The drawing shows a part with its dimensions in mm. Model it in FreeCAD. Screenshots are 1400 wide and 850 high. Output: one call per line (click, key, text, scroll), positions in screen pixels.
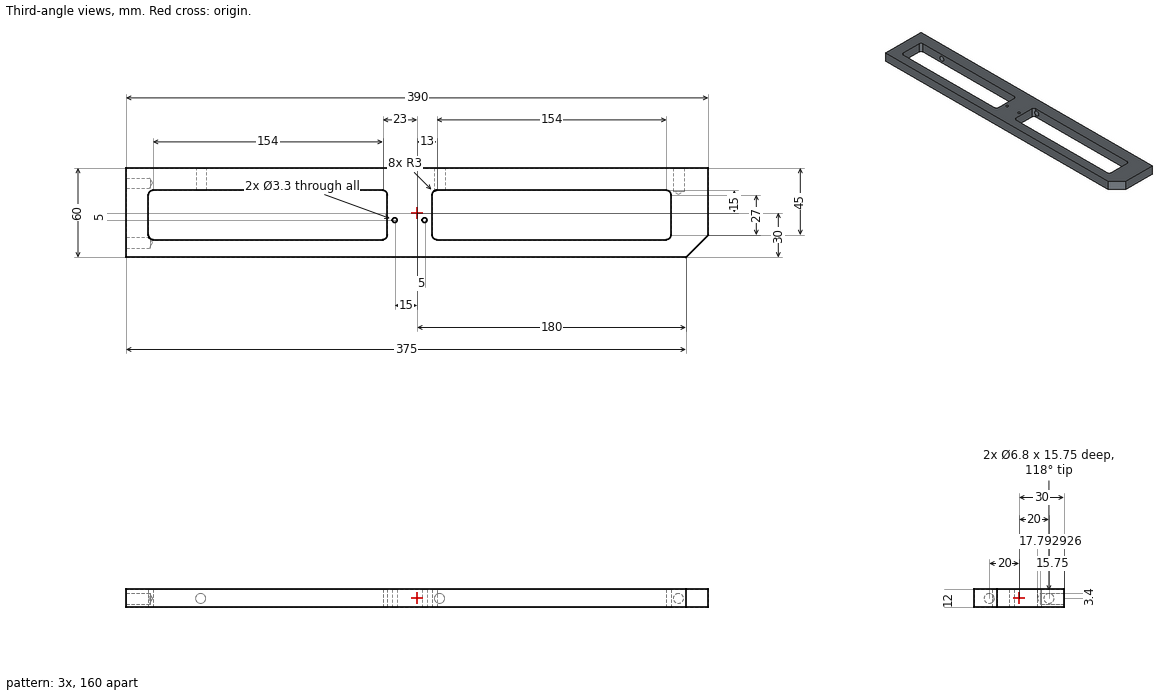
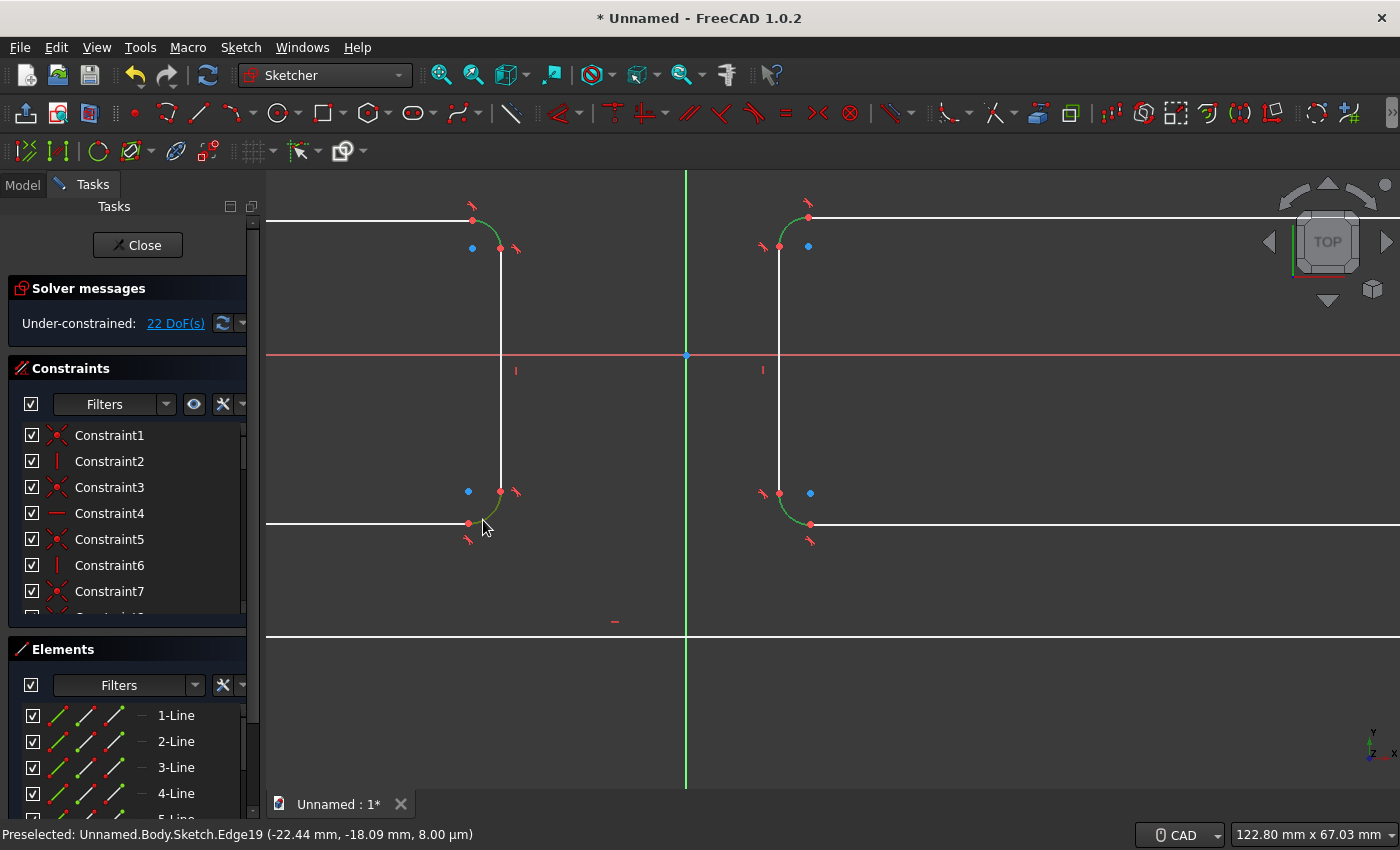
scroll(784, 511, down, 8)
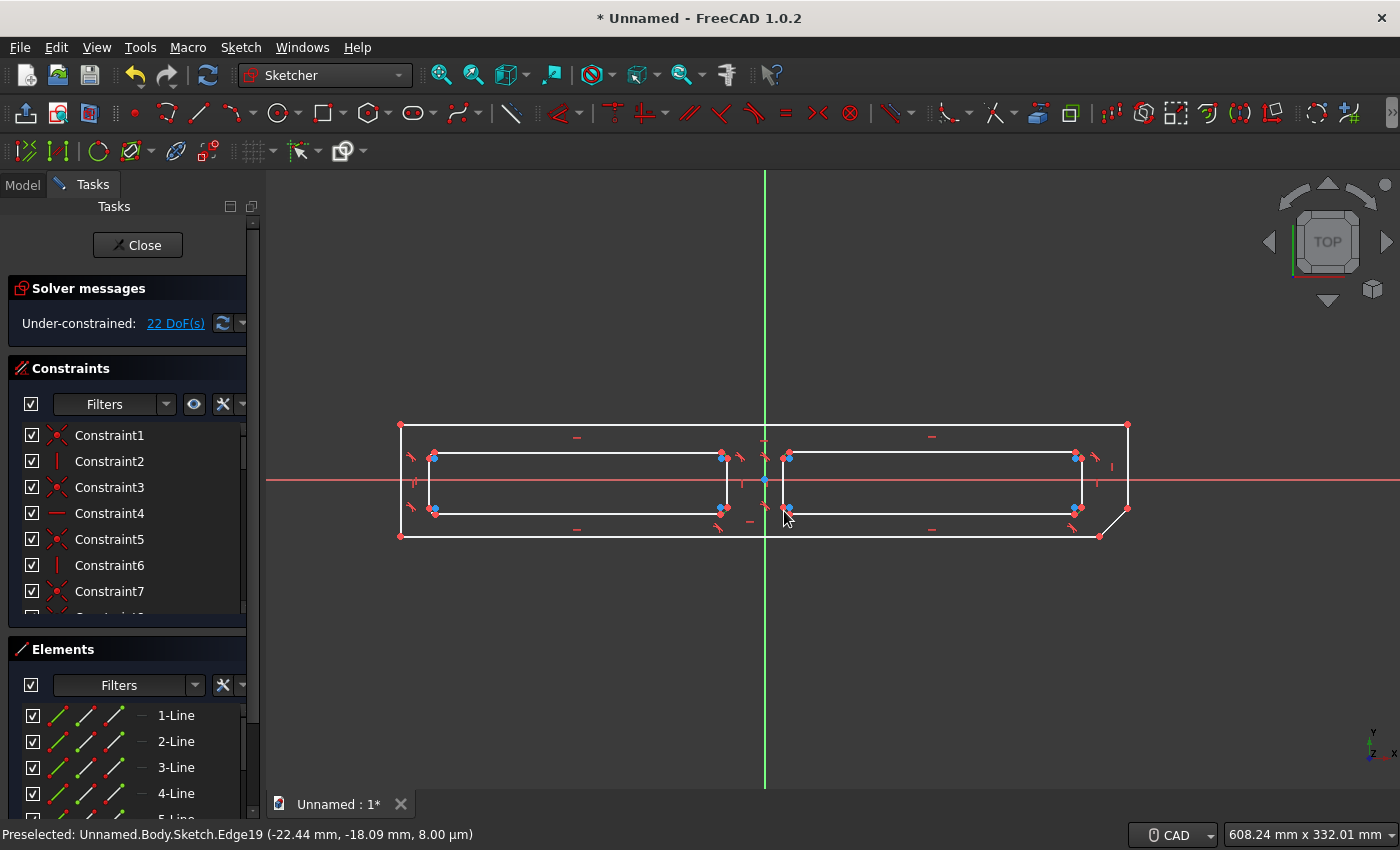
scroll(430, 511, up, 8)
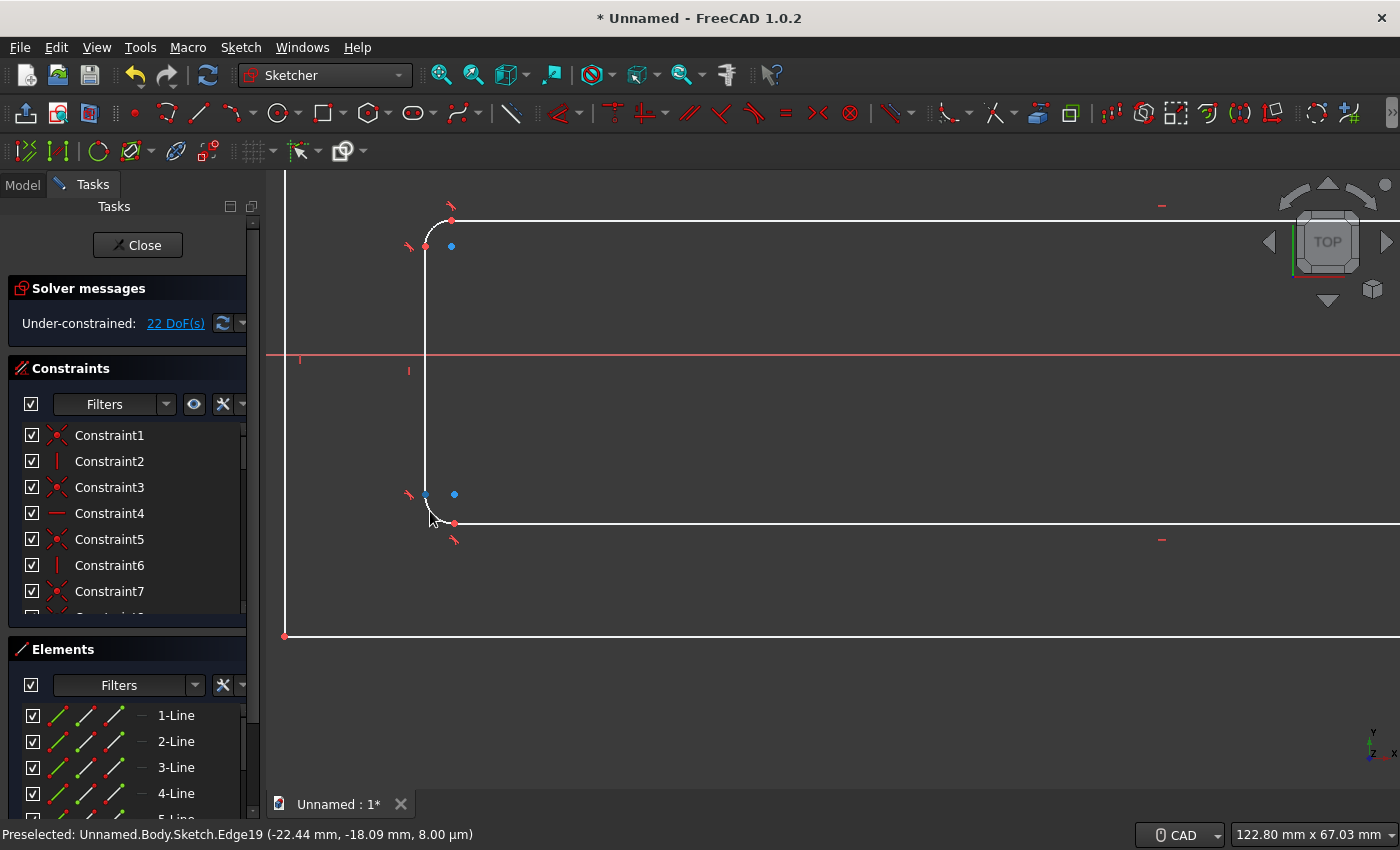
click(428, 508)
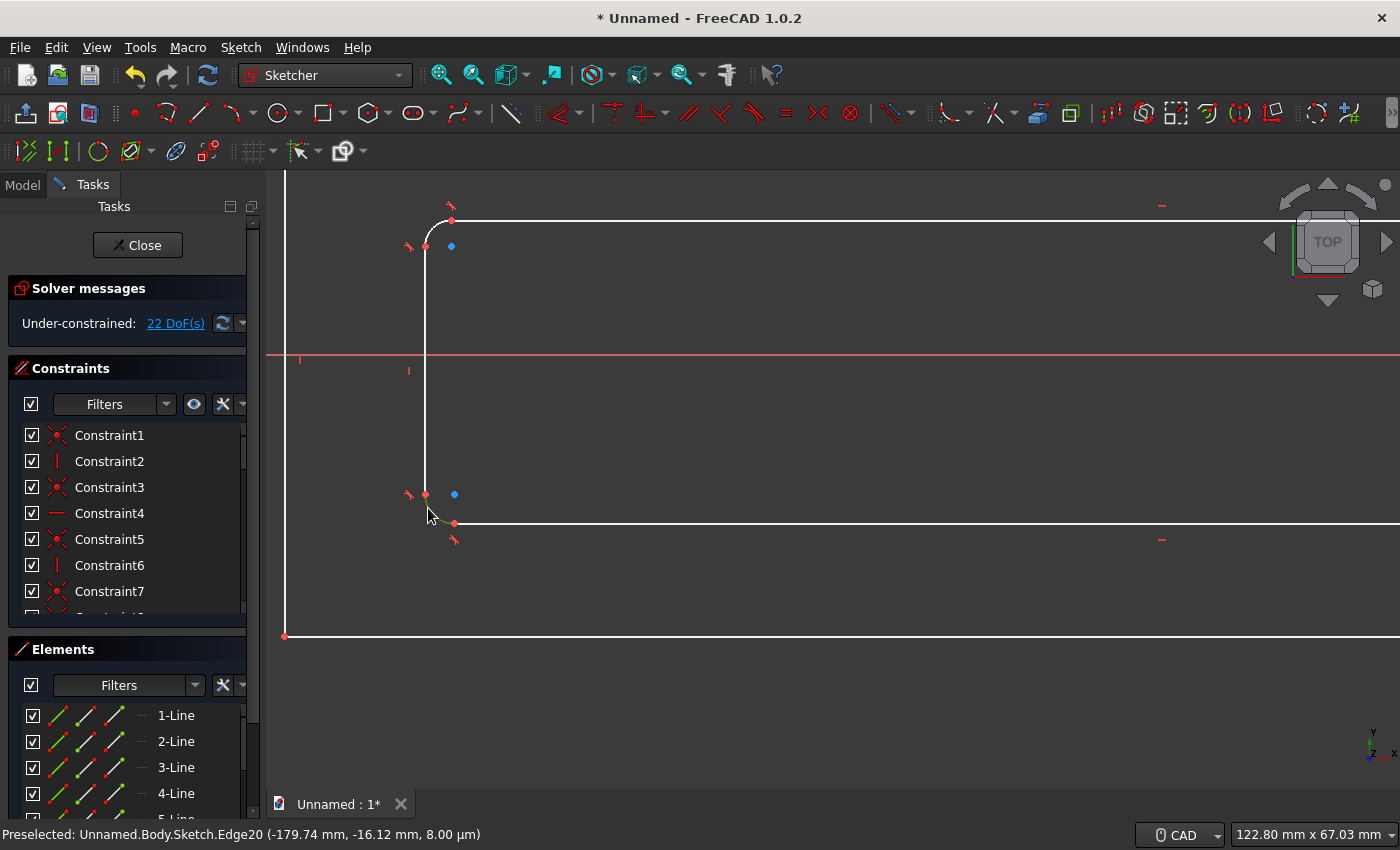
click(439, 223)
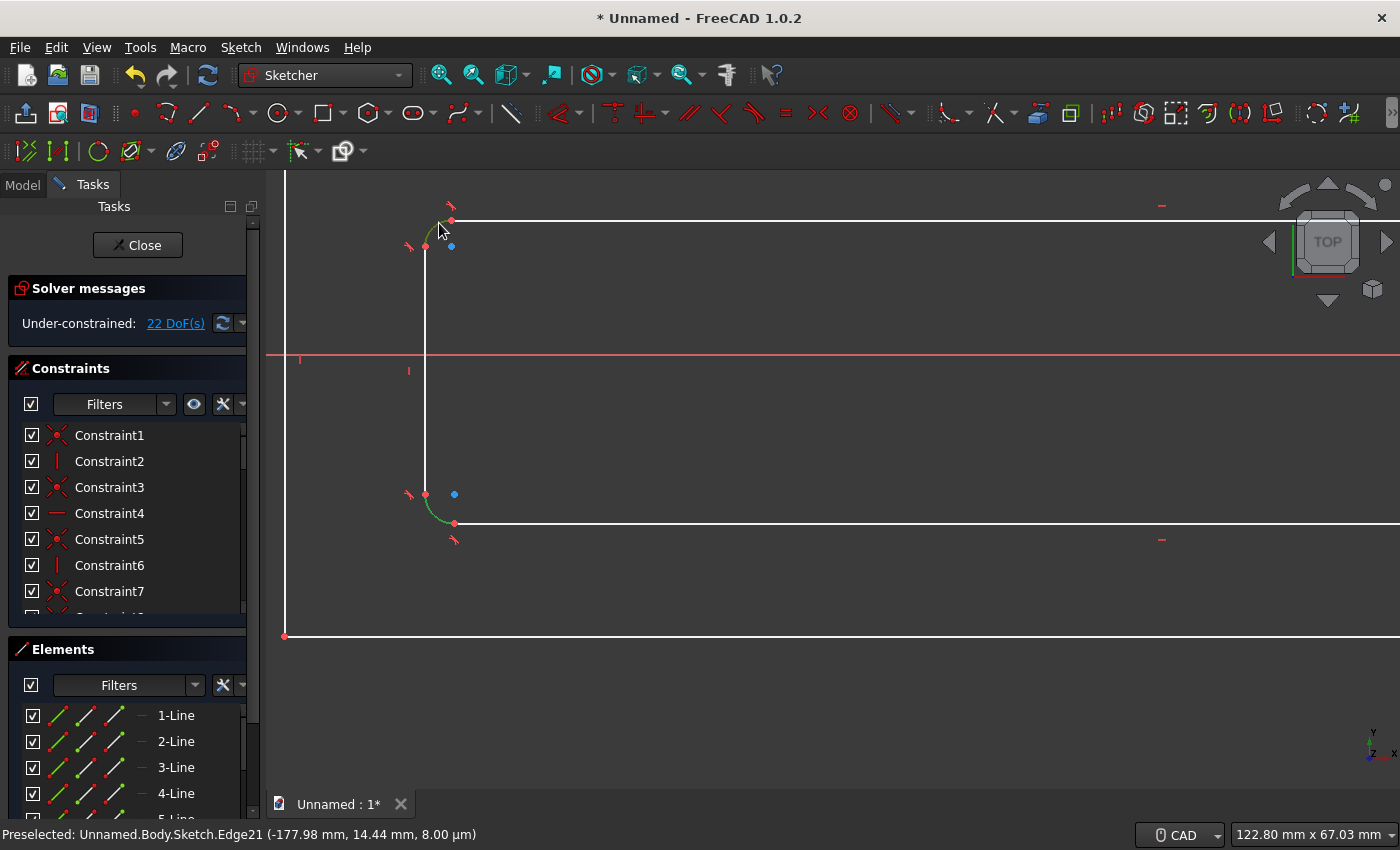
key(e)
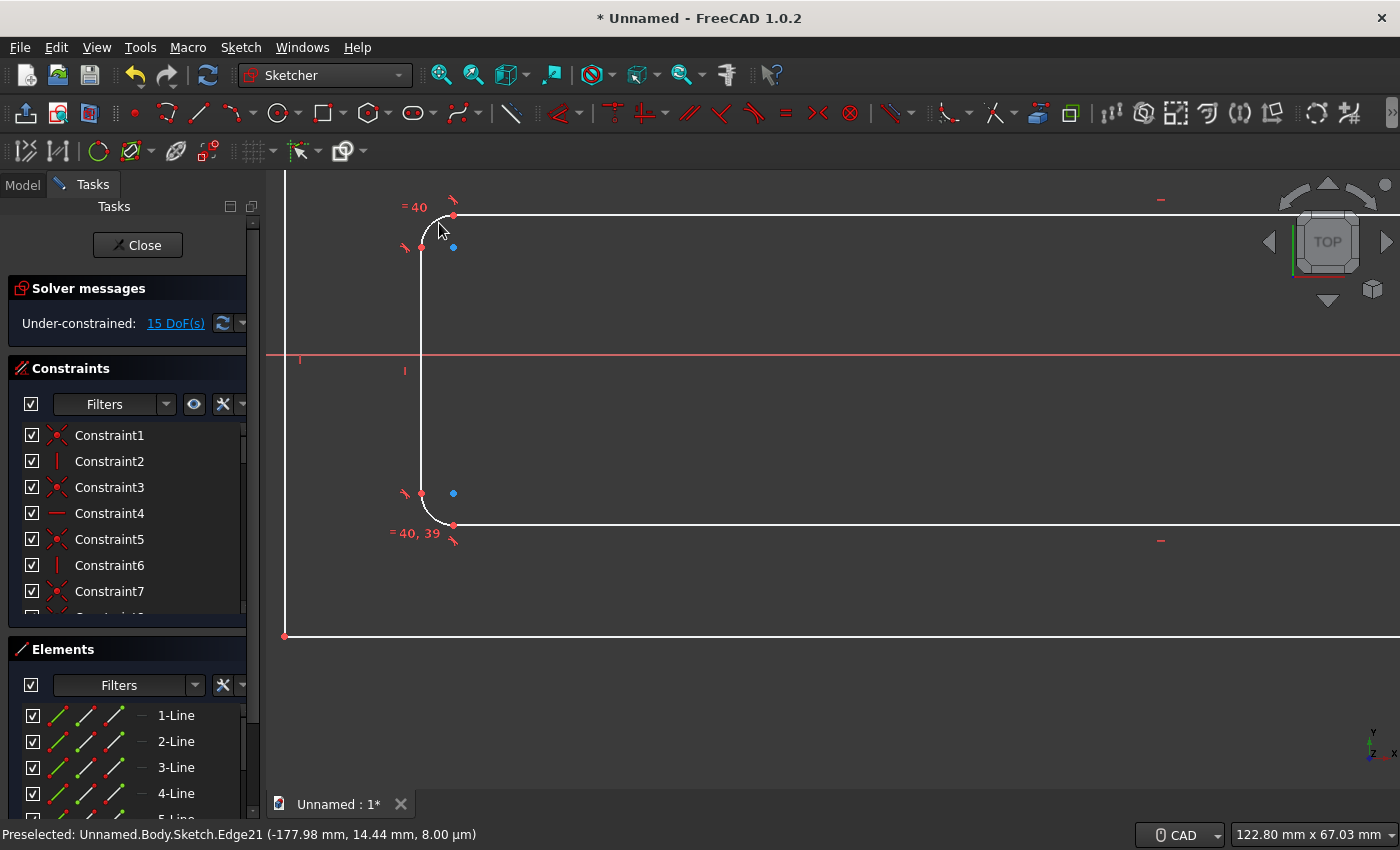
scroll(430, 511, down, 8)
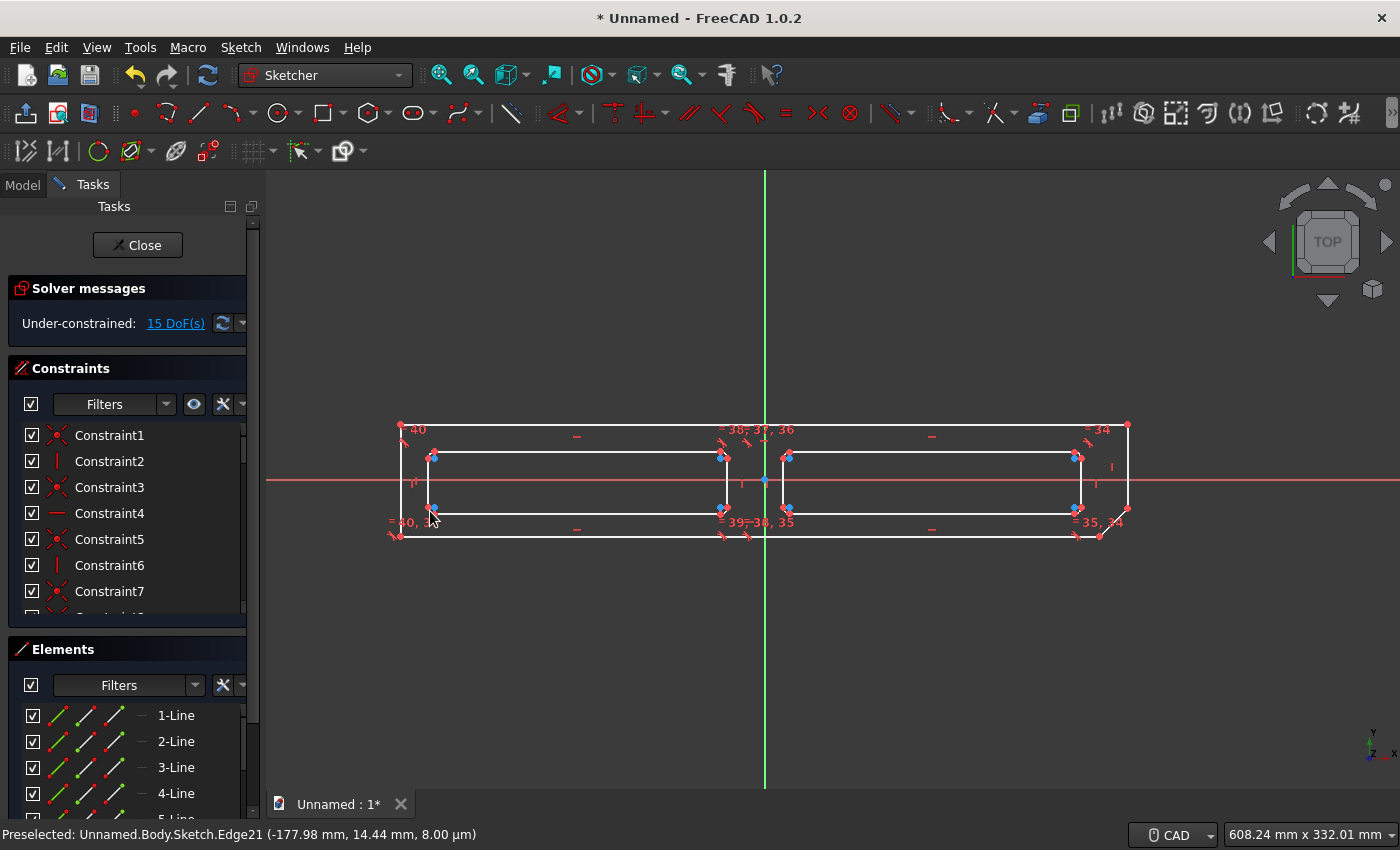
scroll(1081, 456, up, 10)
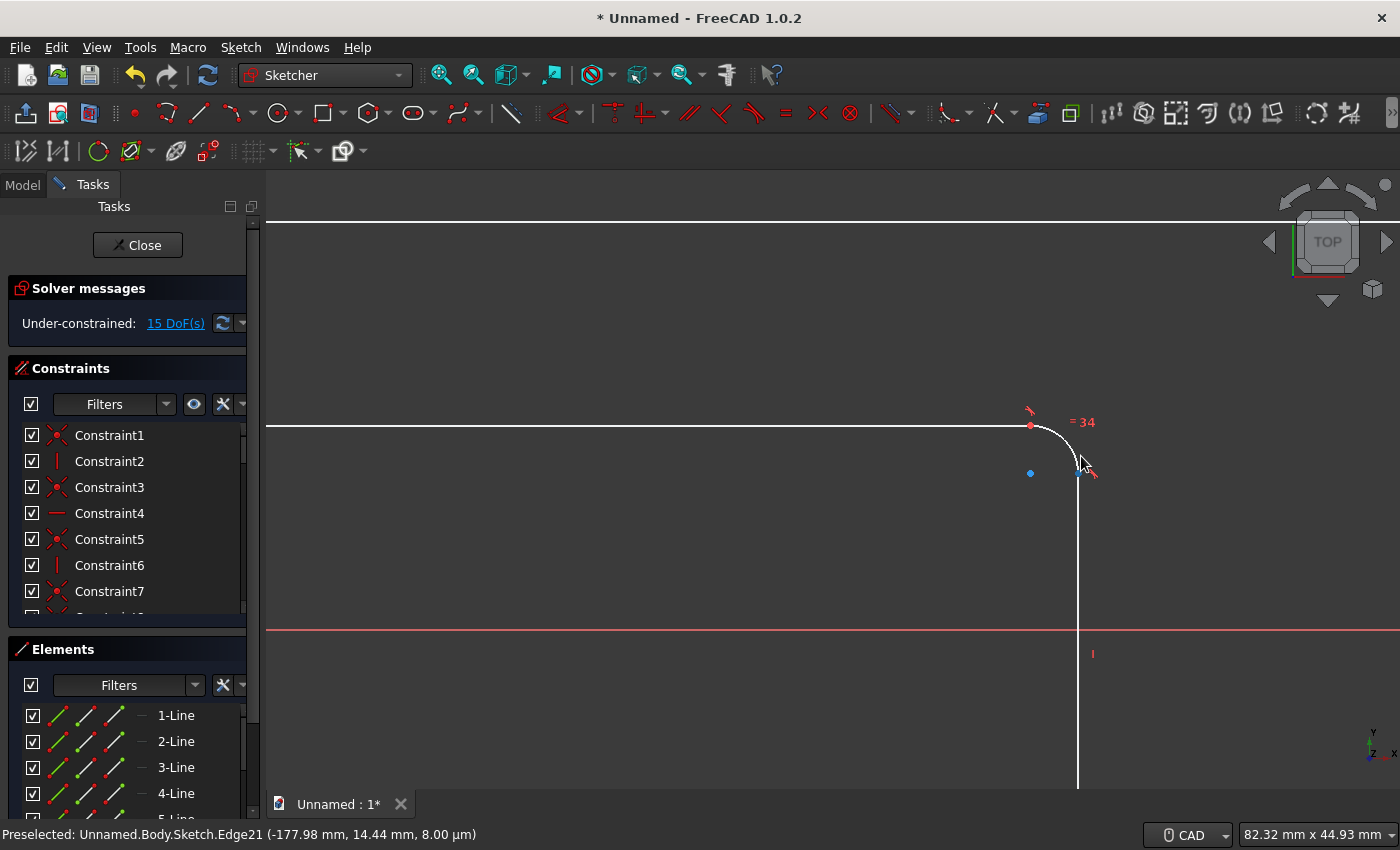
click(1073, 452)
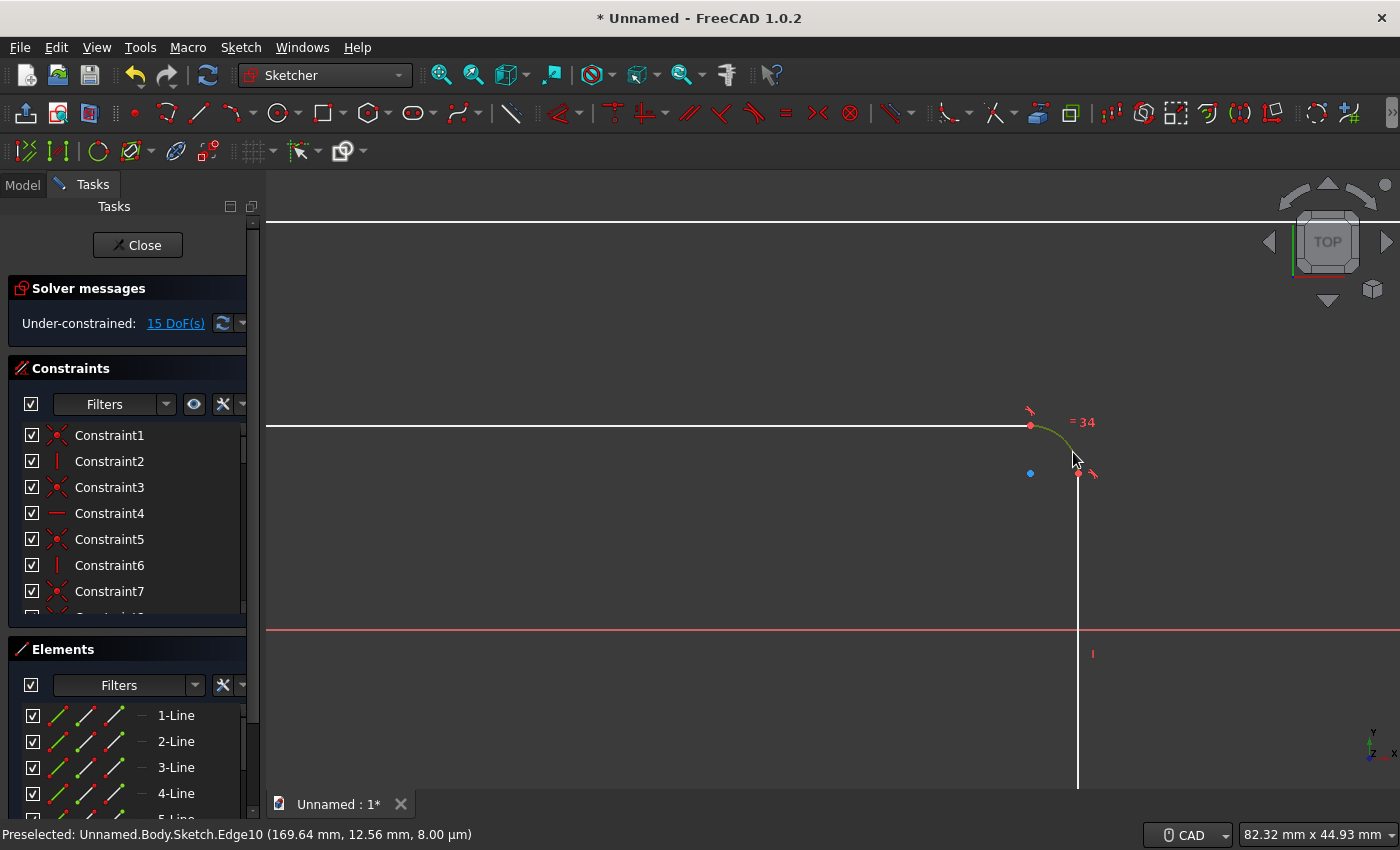
key(k)
key(r)